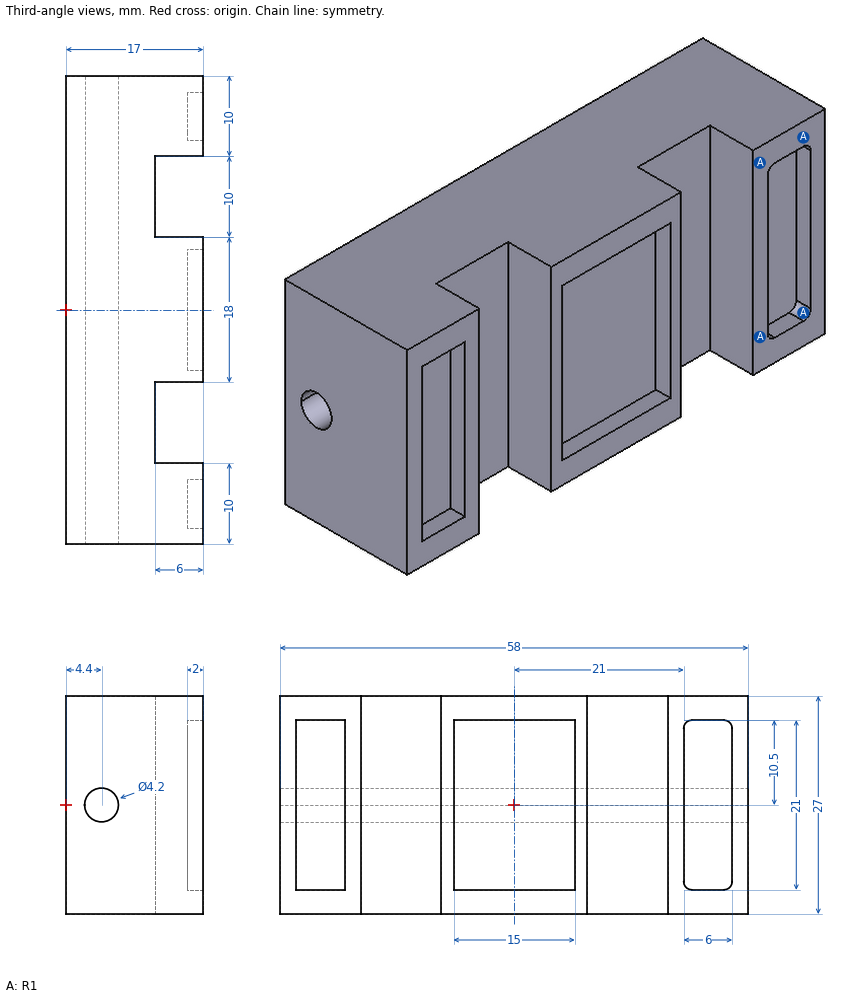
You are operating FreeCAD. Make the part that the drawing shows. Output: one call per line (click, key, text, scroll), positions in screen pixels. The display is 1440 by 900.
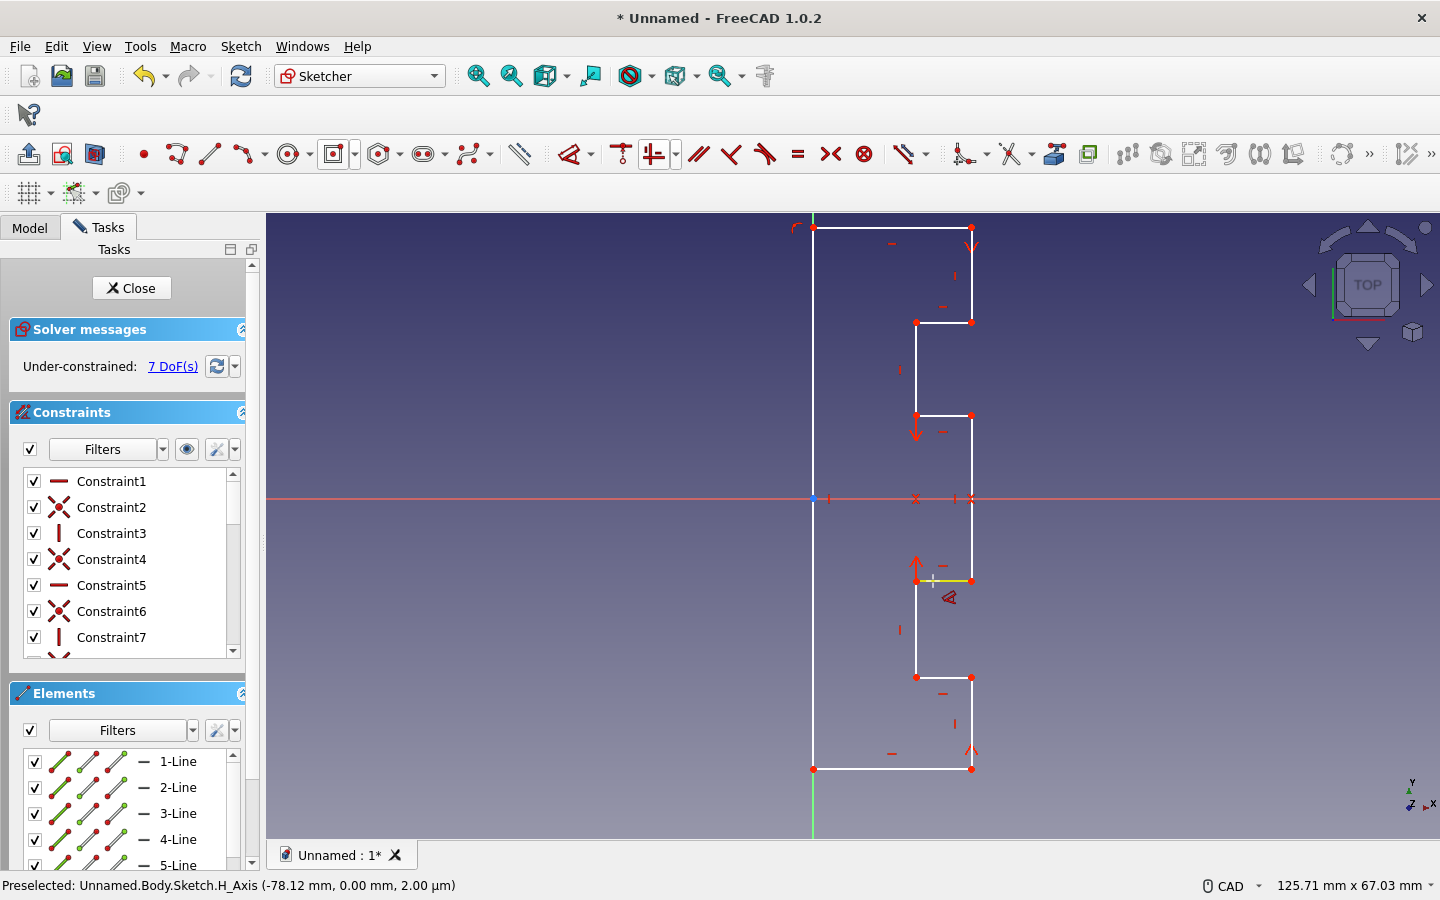
click(933, 581)
click(944, 615)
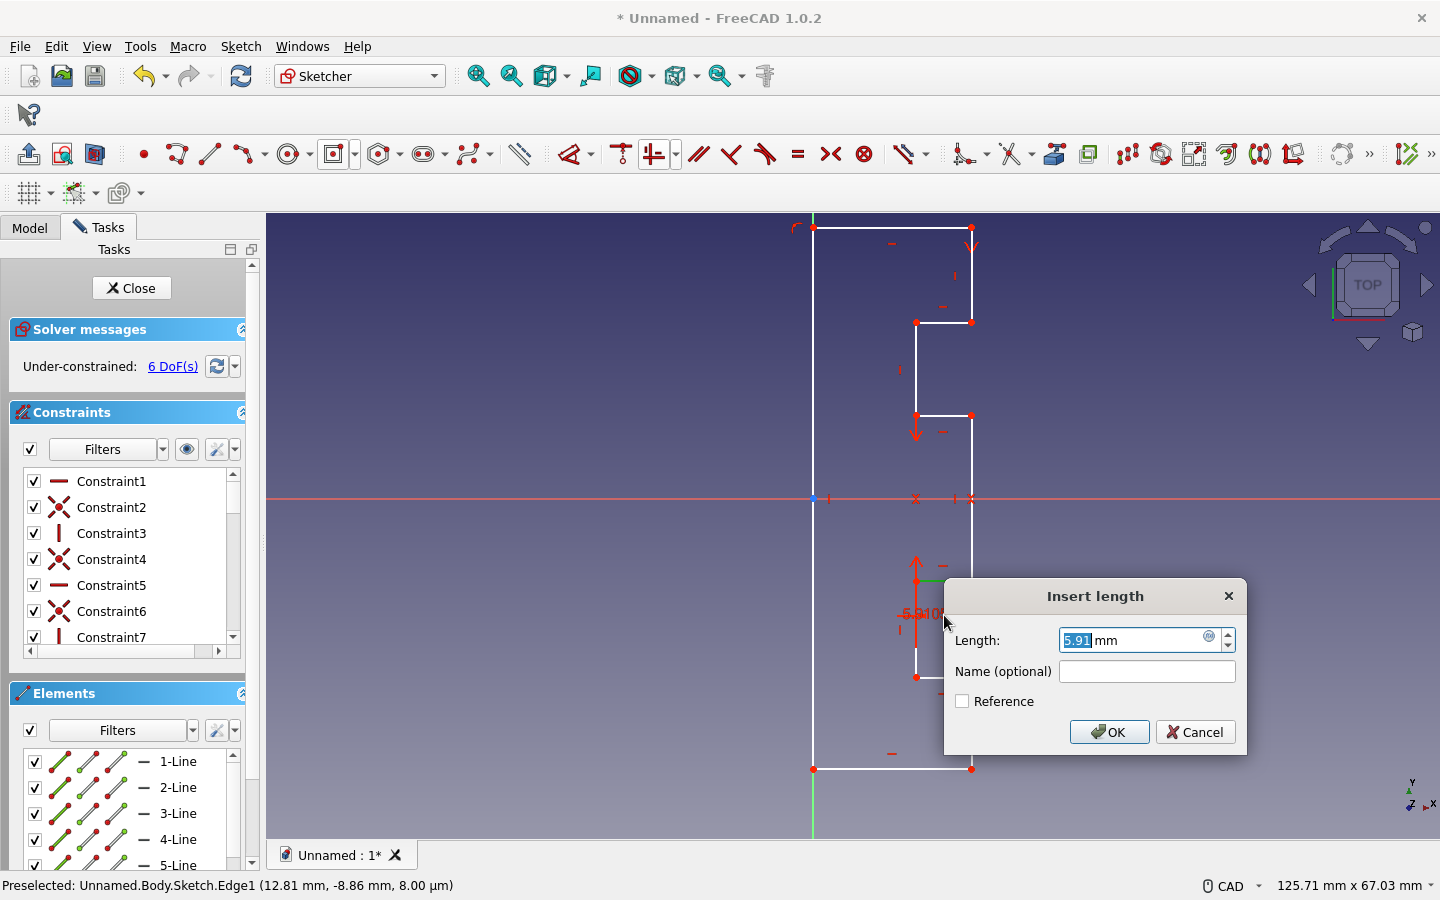
text(6)
key(Return)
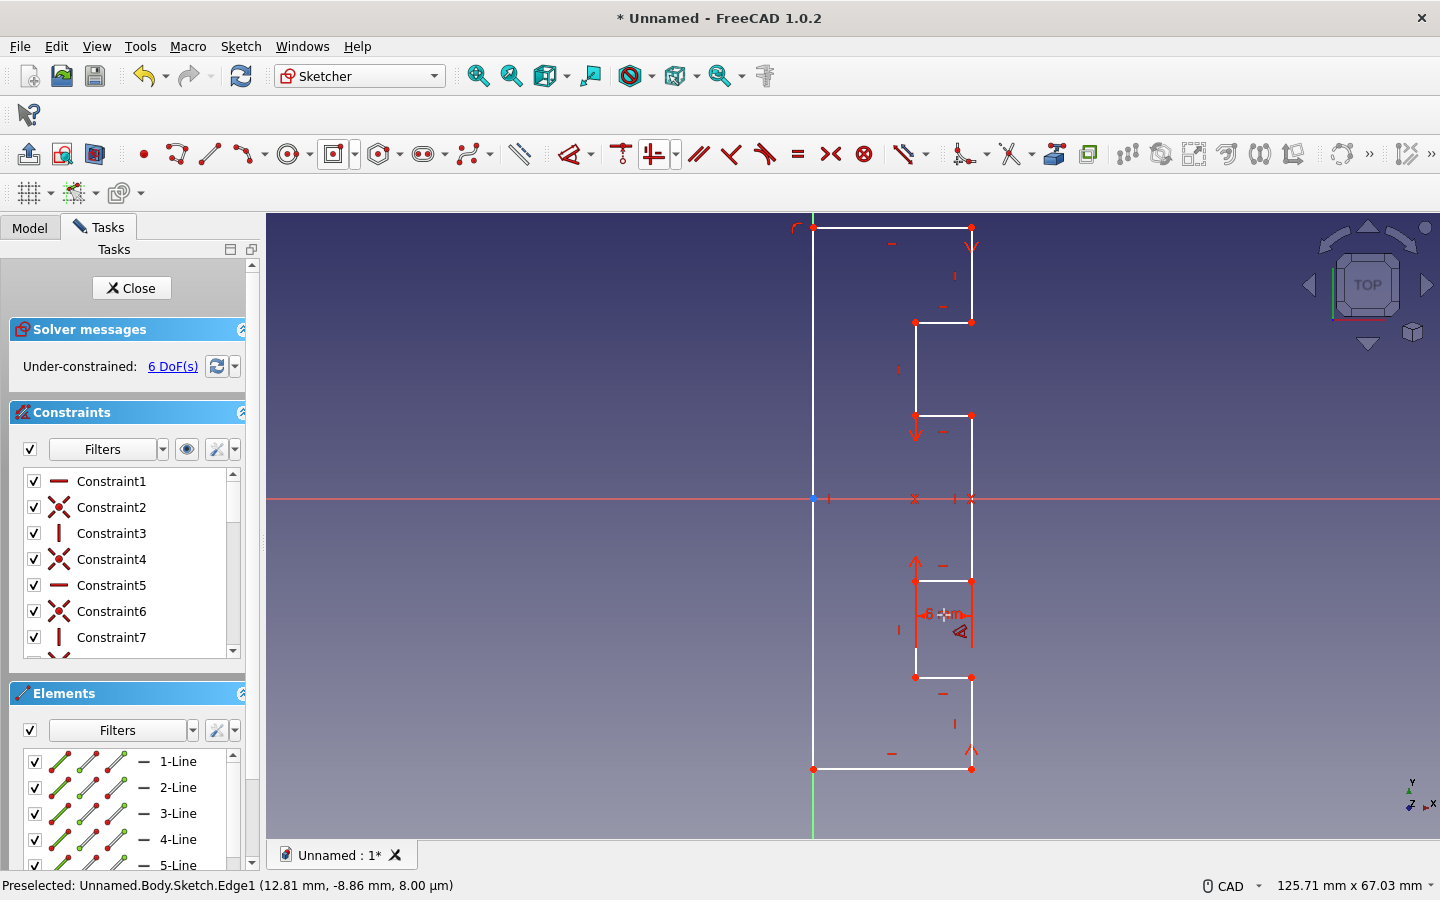
click(932, 323)
click(944, 289)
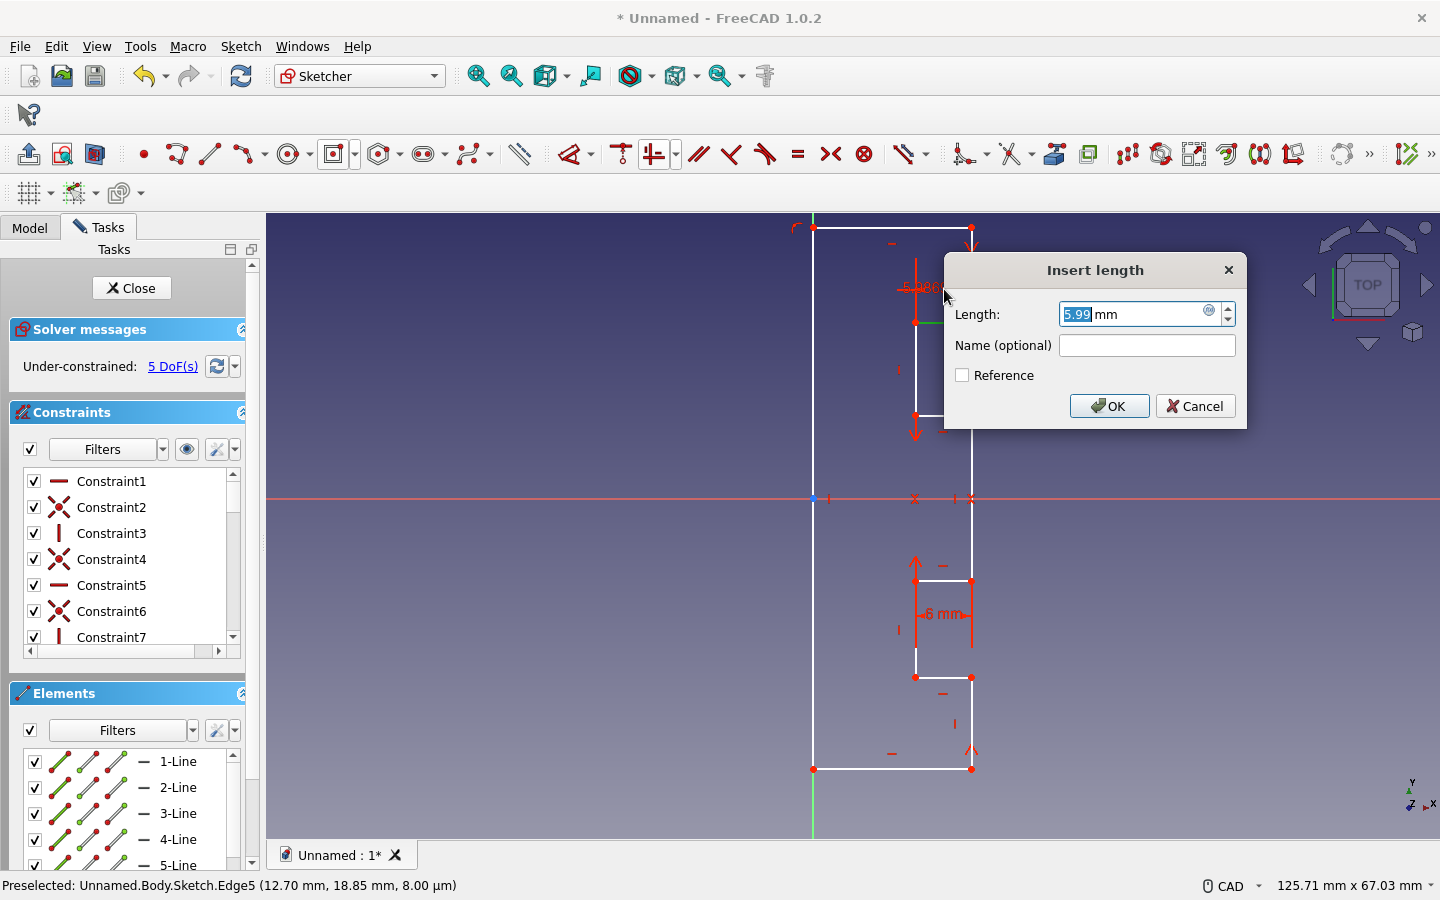
text(6)
key(Return)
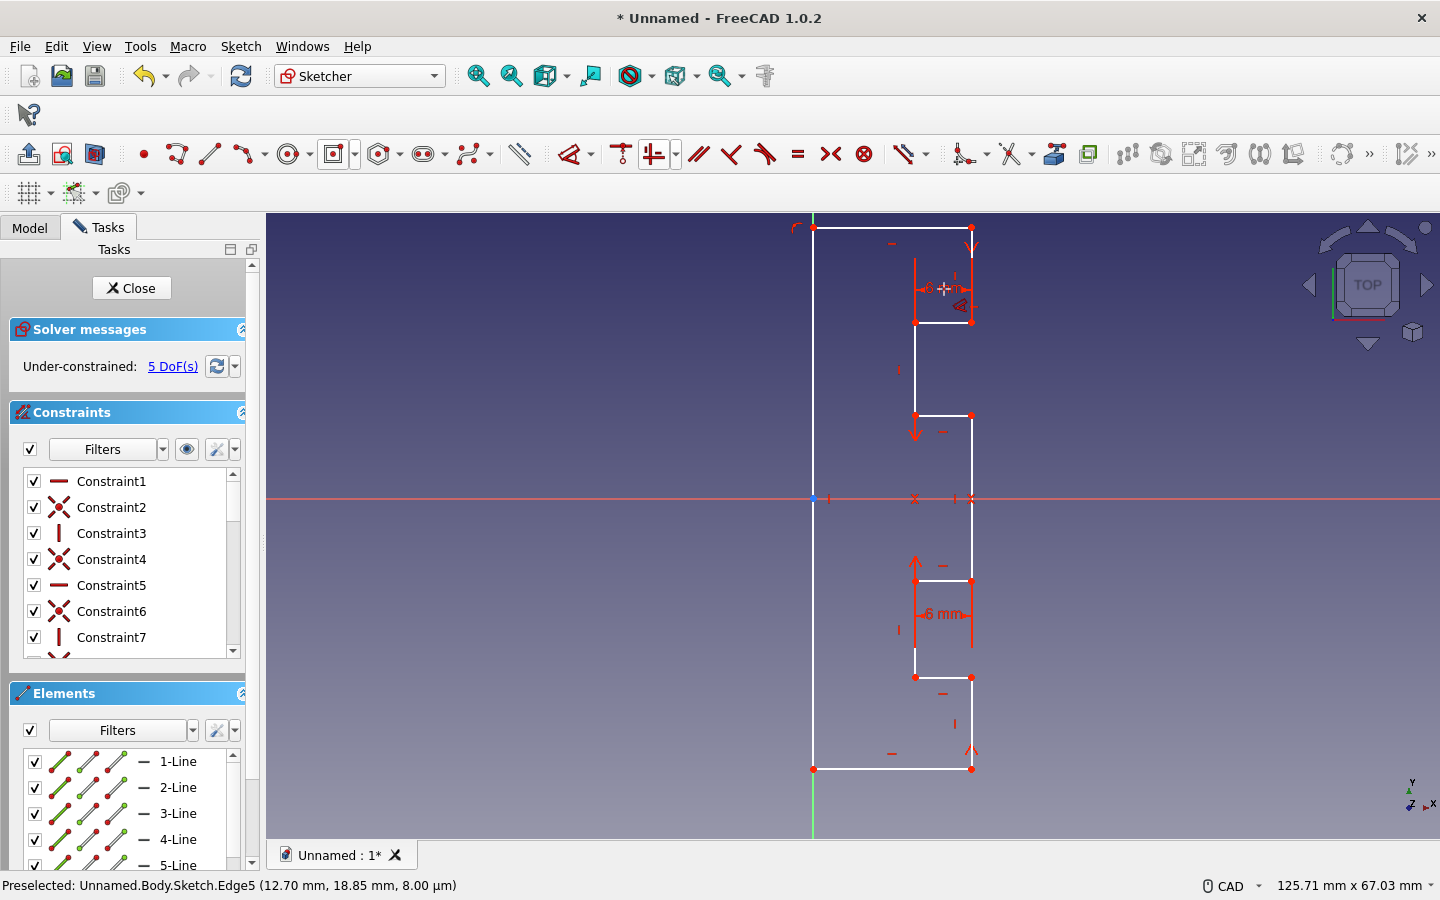
click(972, 532)
click(1006, 461)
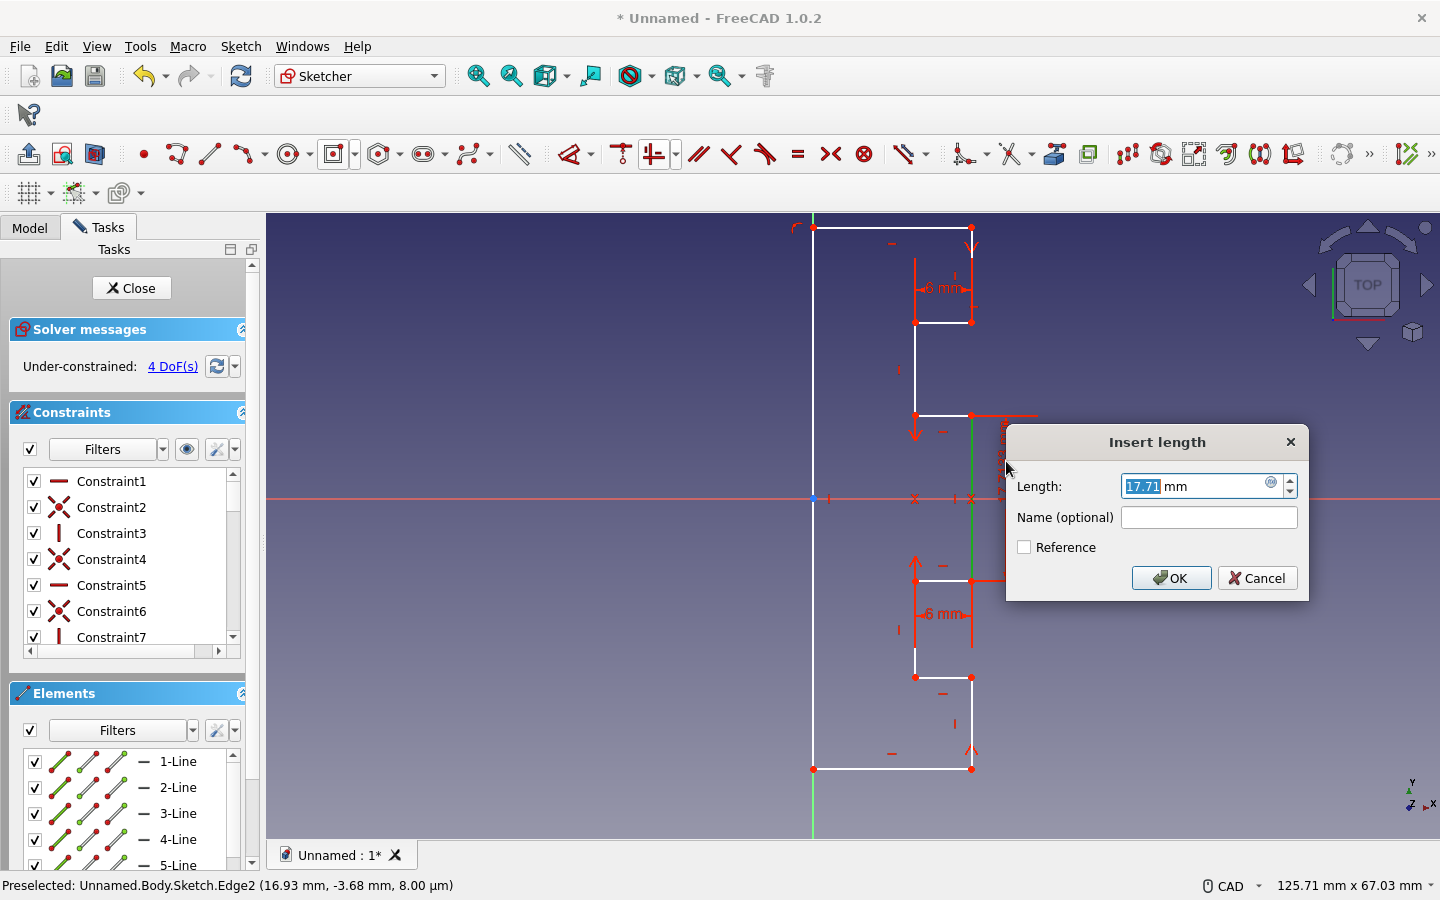
text(18)
key(Return)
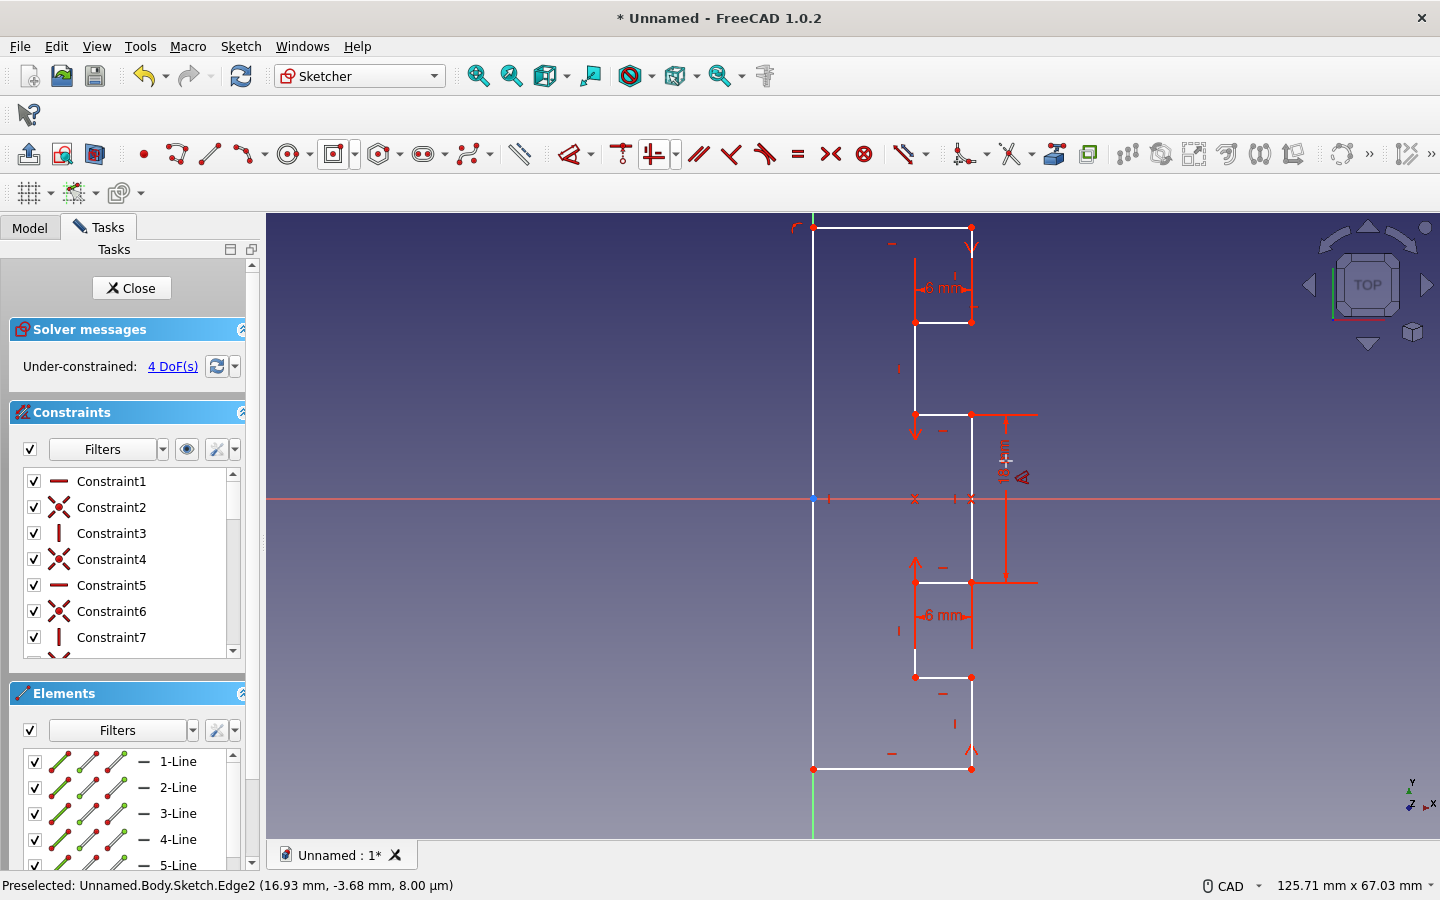
click(915, 387)
click(949, 369)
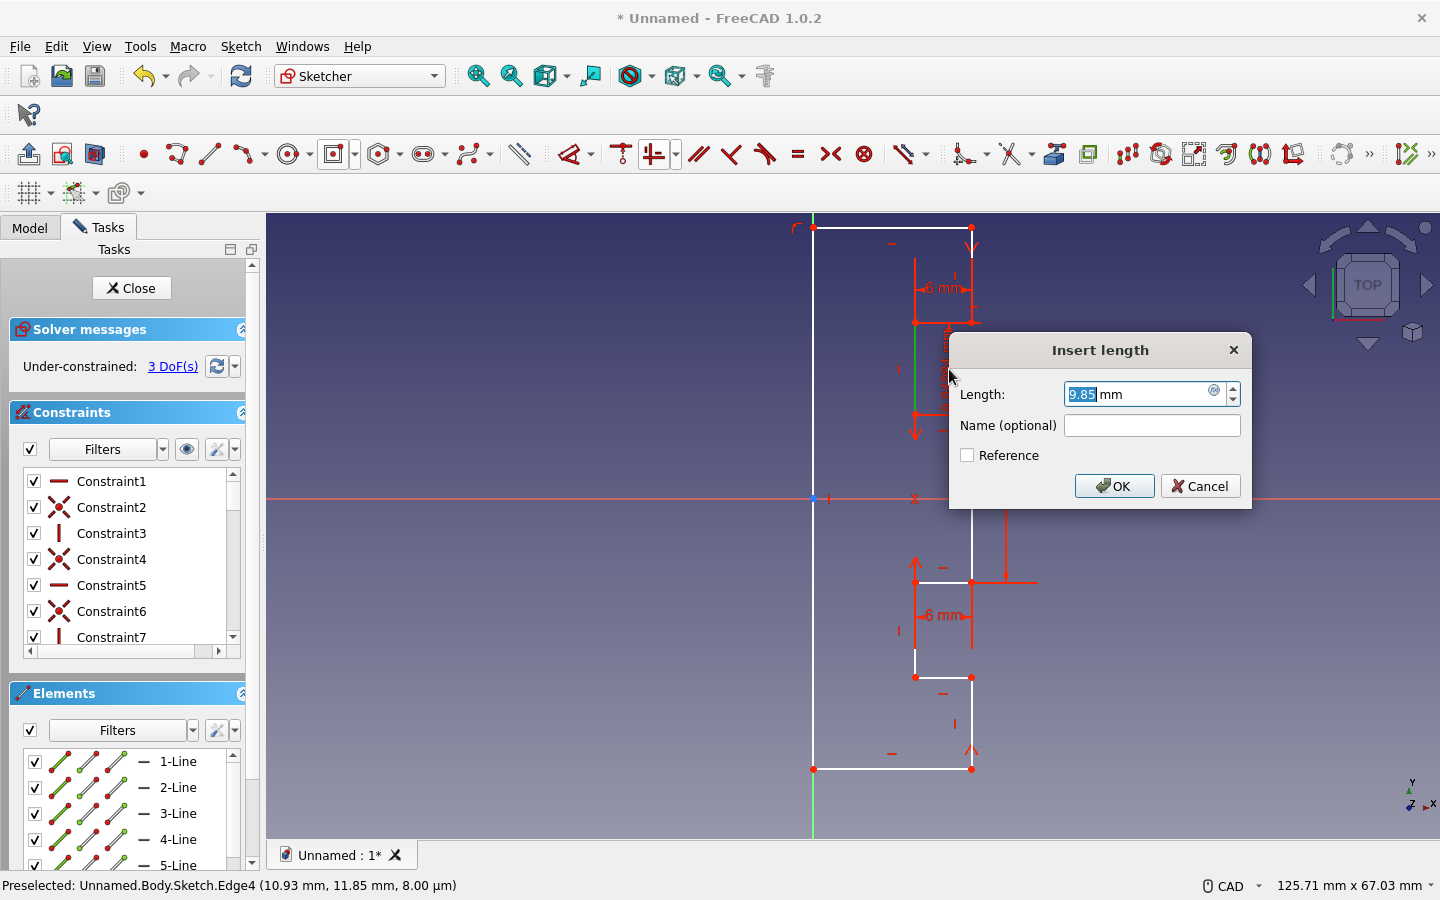
text(10)
key(Return)